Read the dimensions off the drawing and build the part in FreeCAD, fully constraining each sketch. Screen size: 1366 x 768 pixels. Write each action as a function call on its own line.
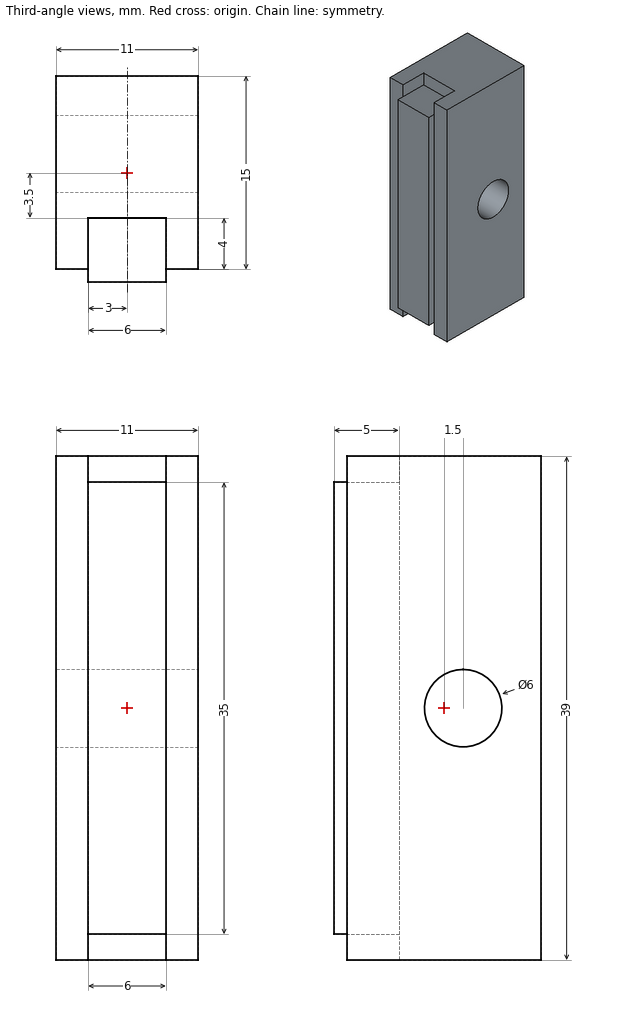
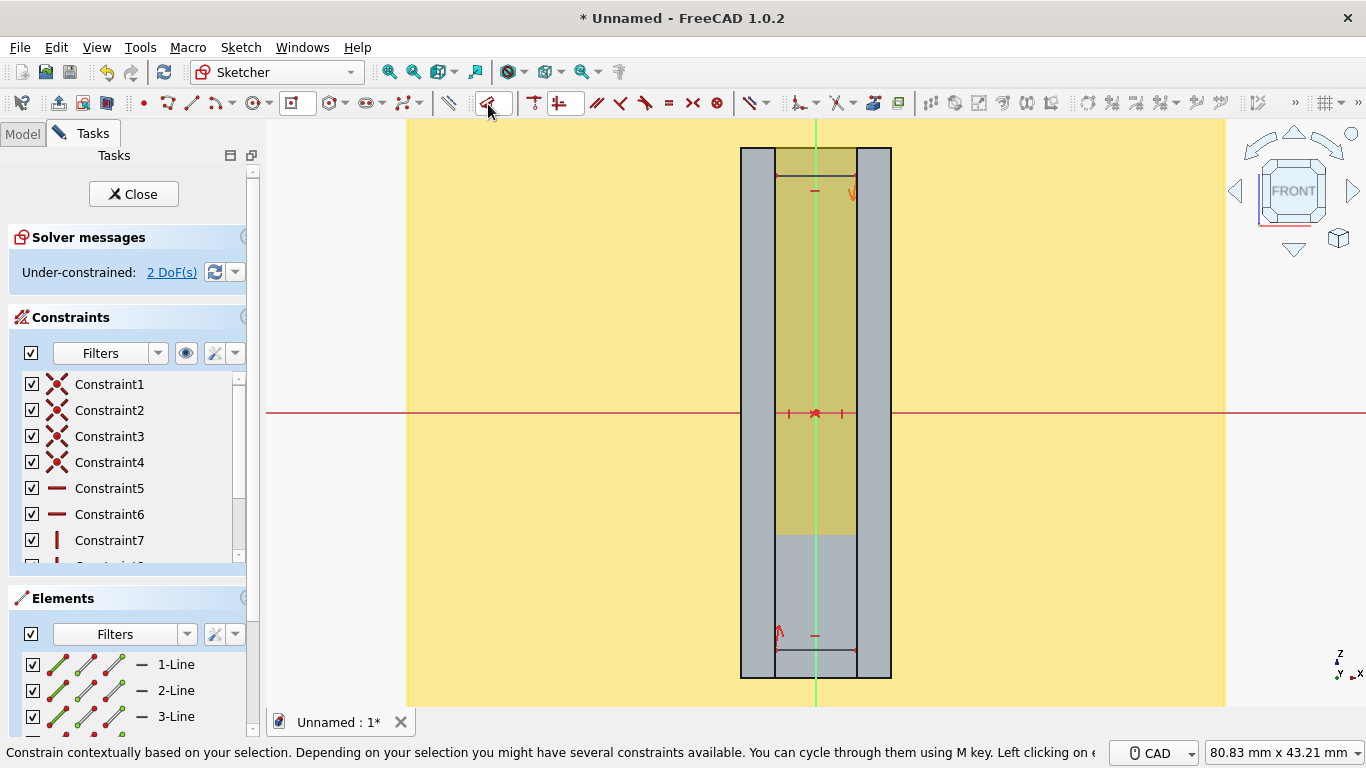
click(800, 650)
click(797, 616)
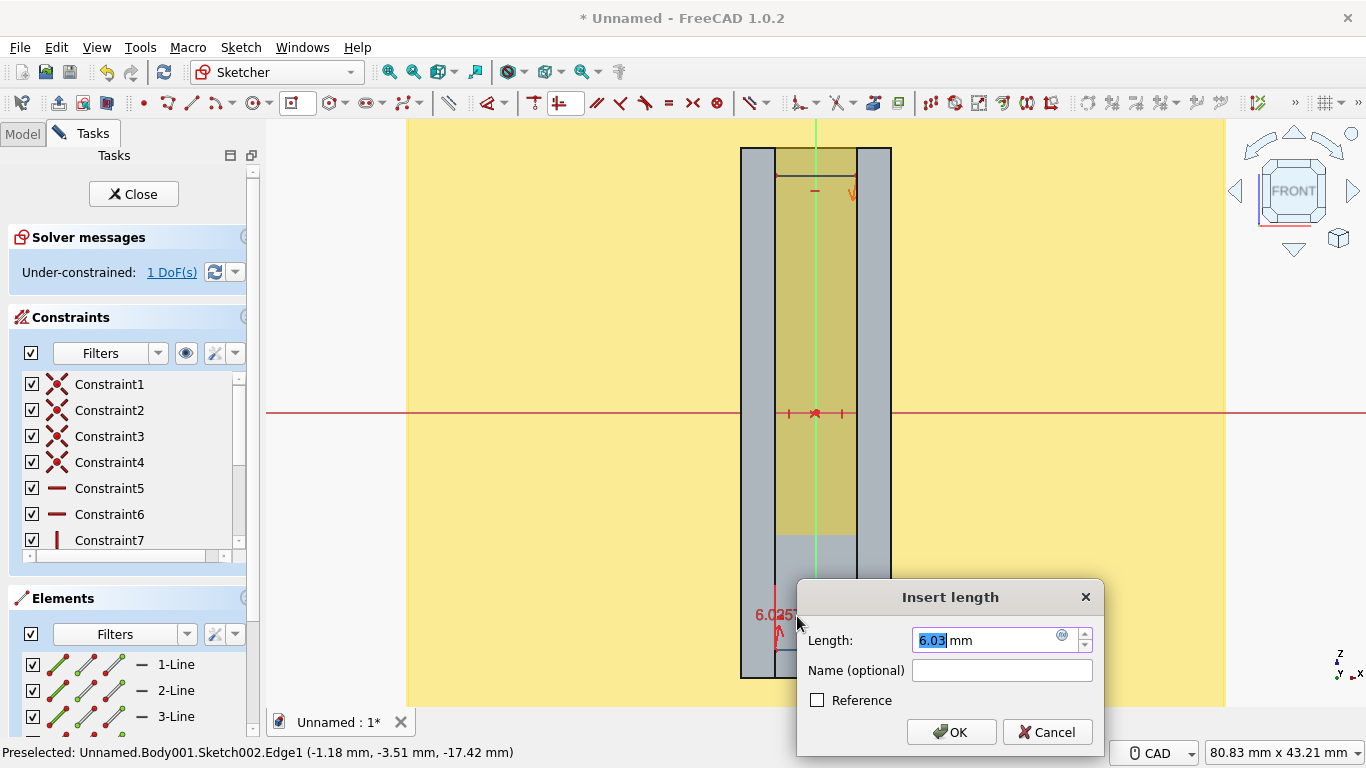
text(6)
key(Return)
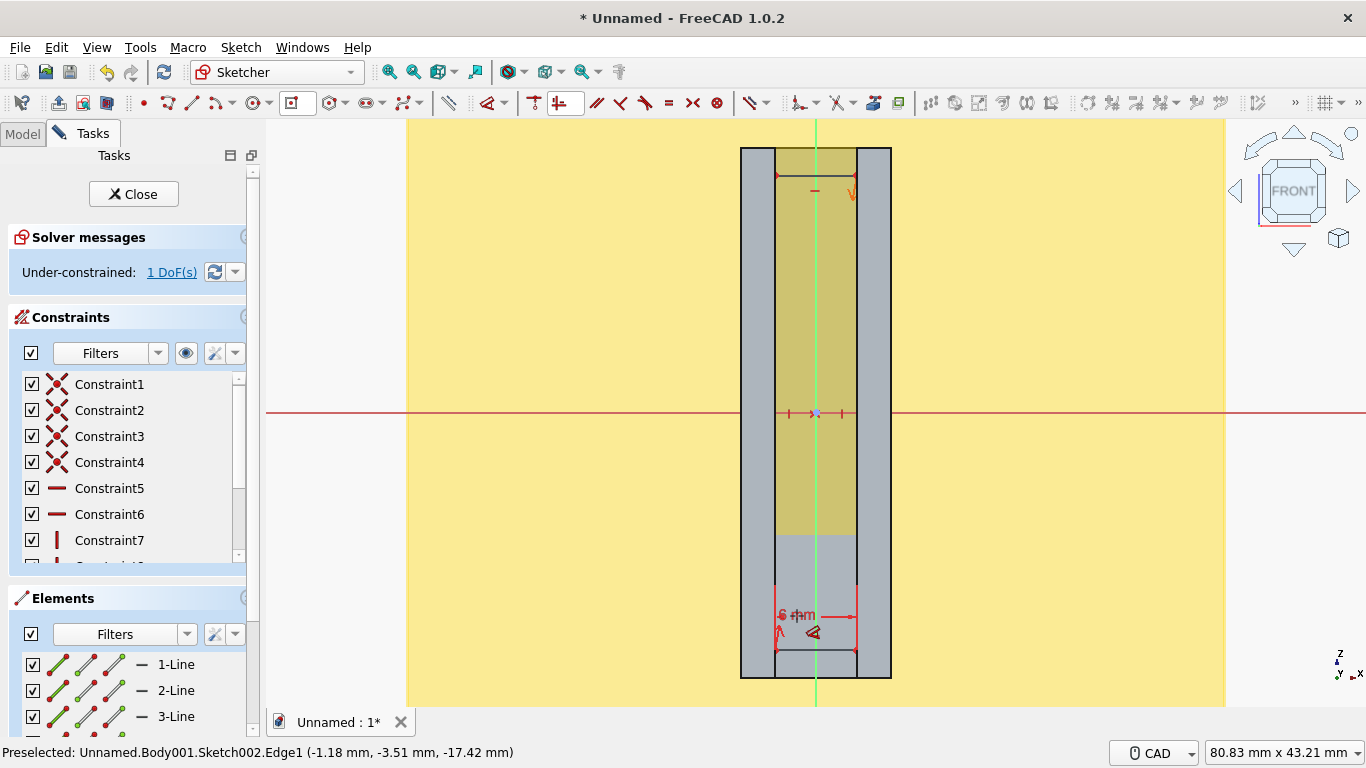
click(857, 508)
click(891, 304)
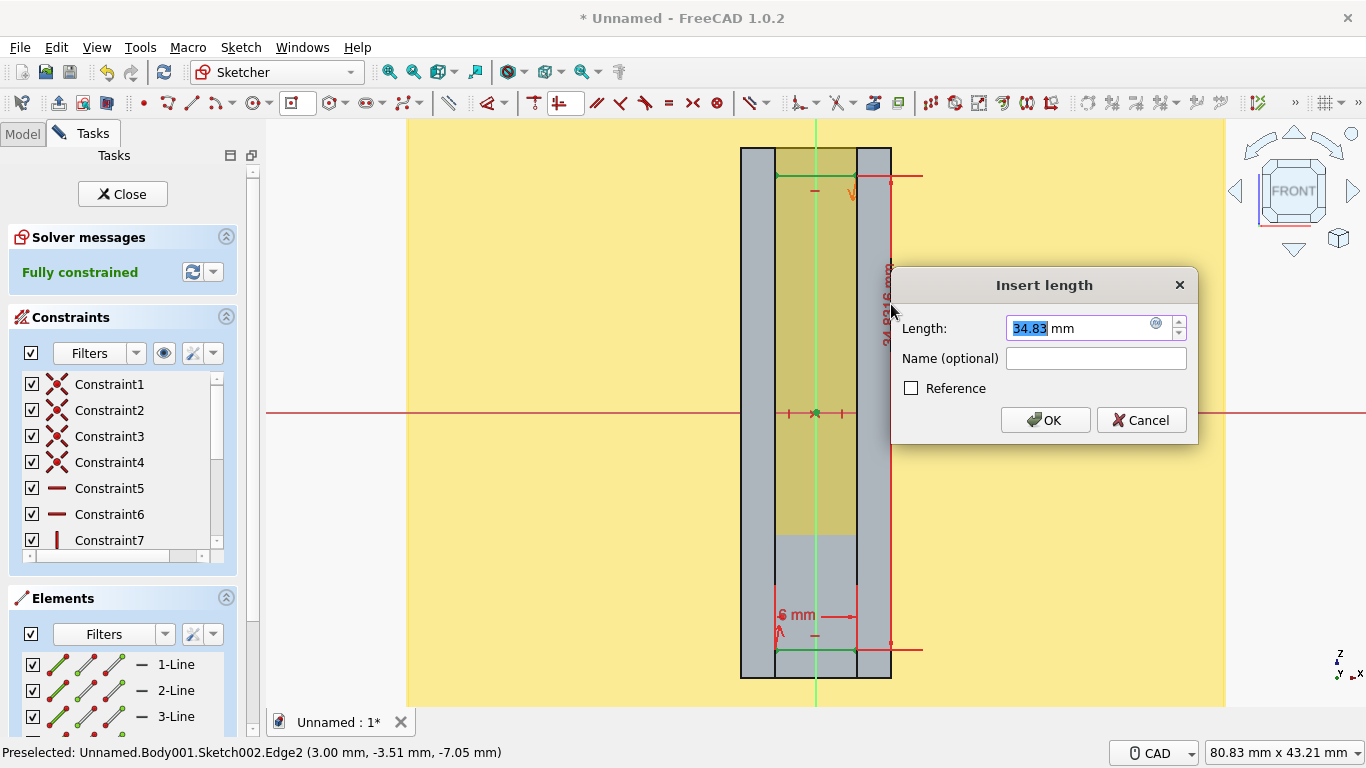
text(35)
key(Return)
key(Escape)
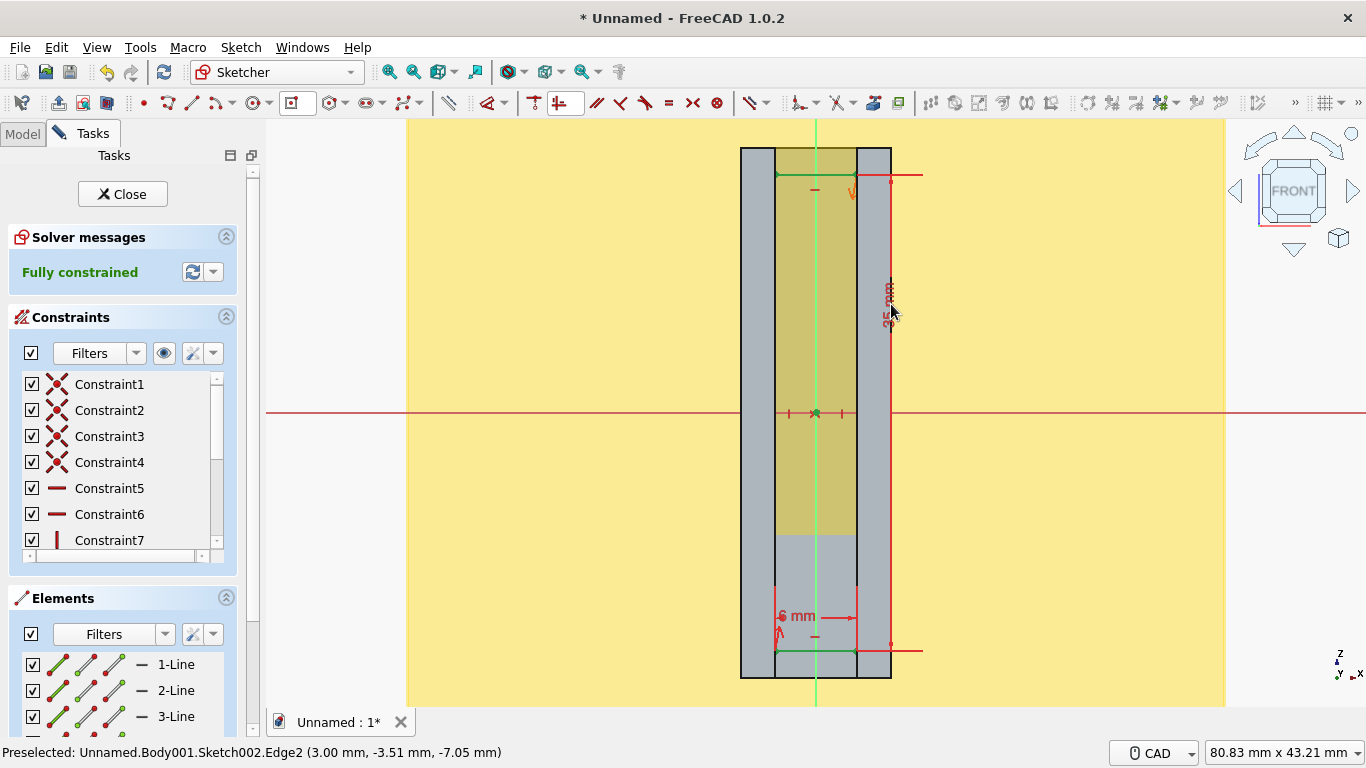
click(123, 194)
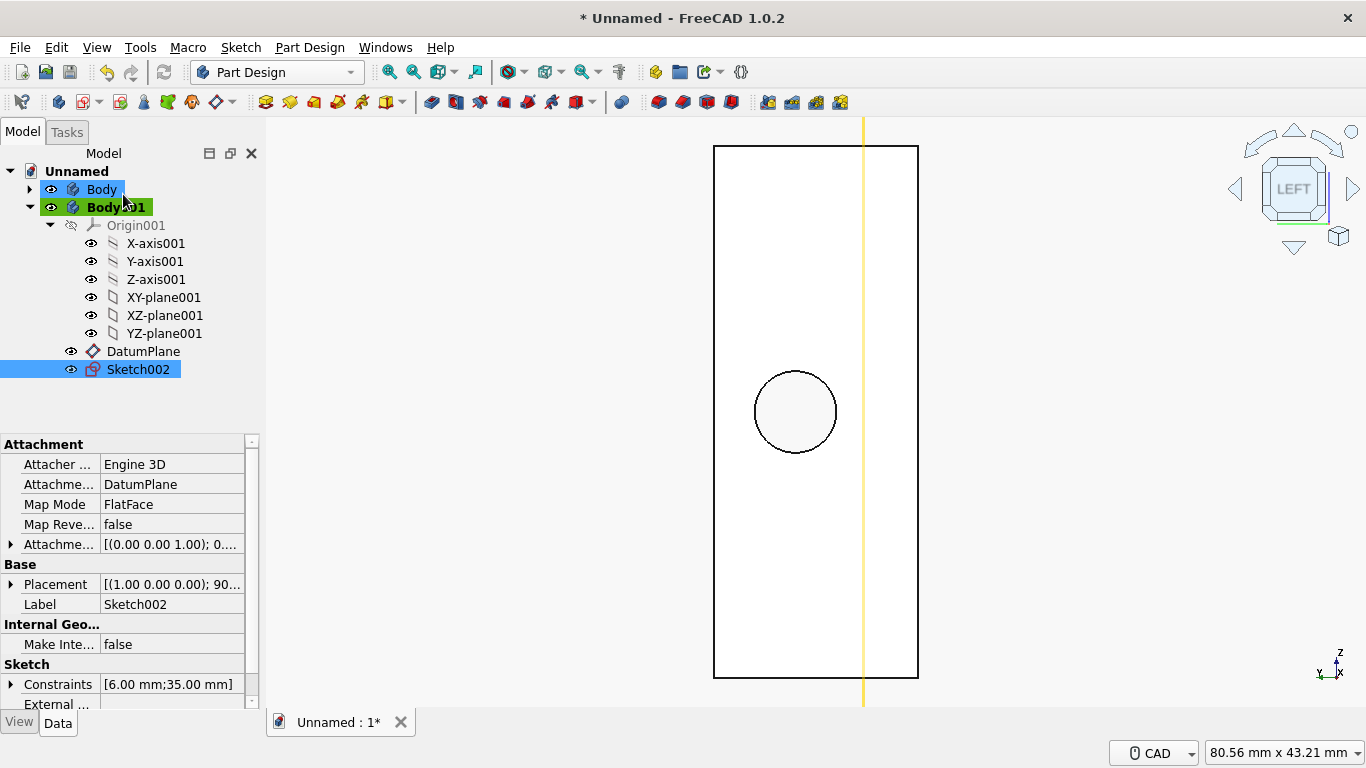
click(266, 102)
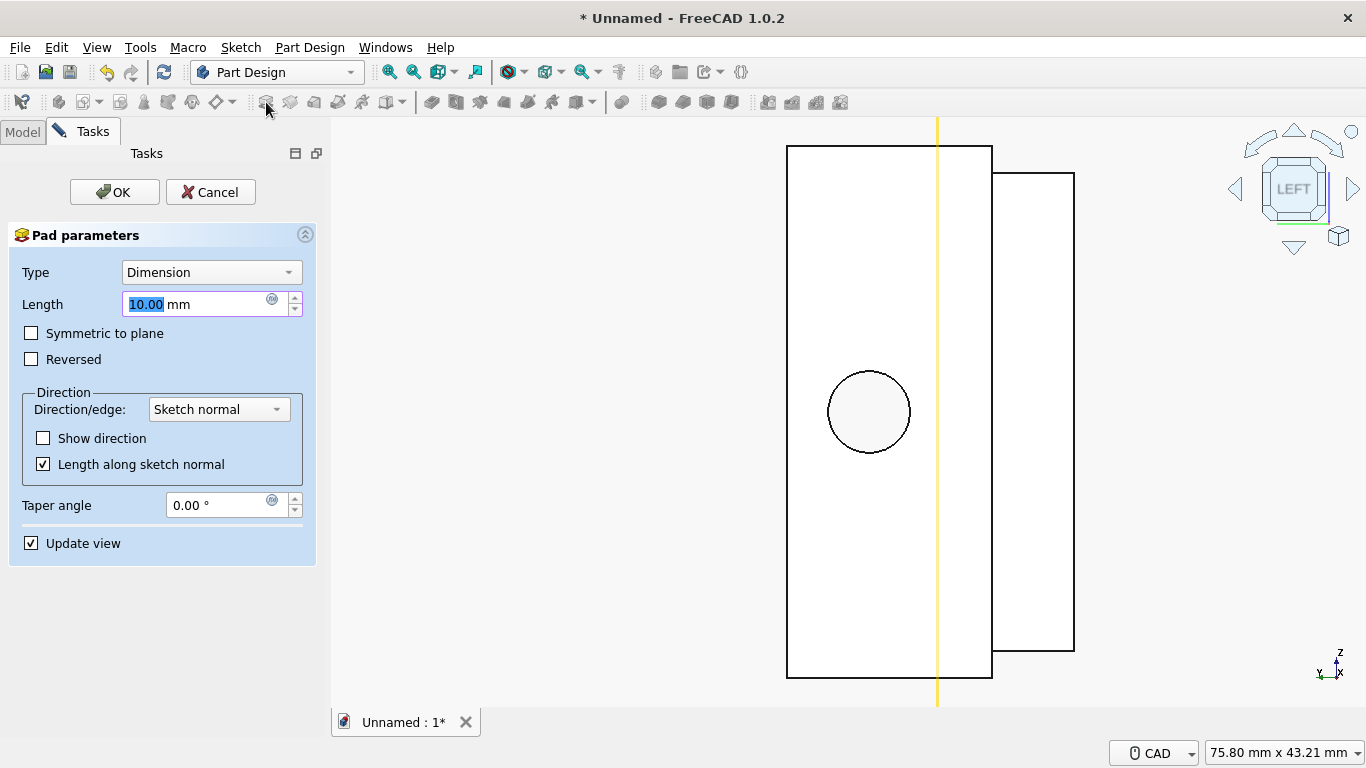
text(5)
key(Tab)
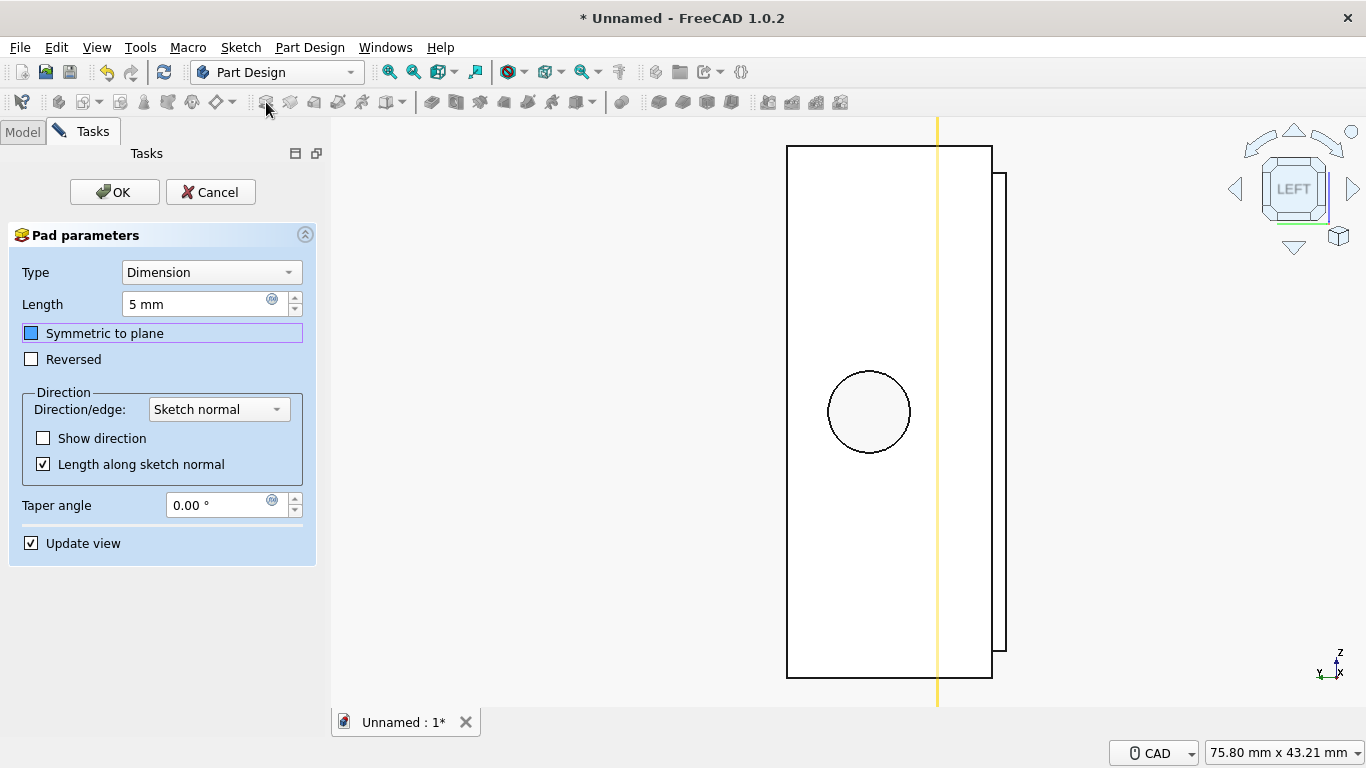
click(115, 192)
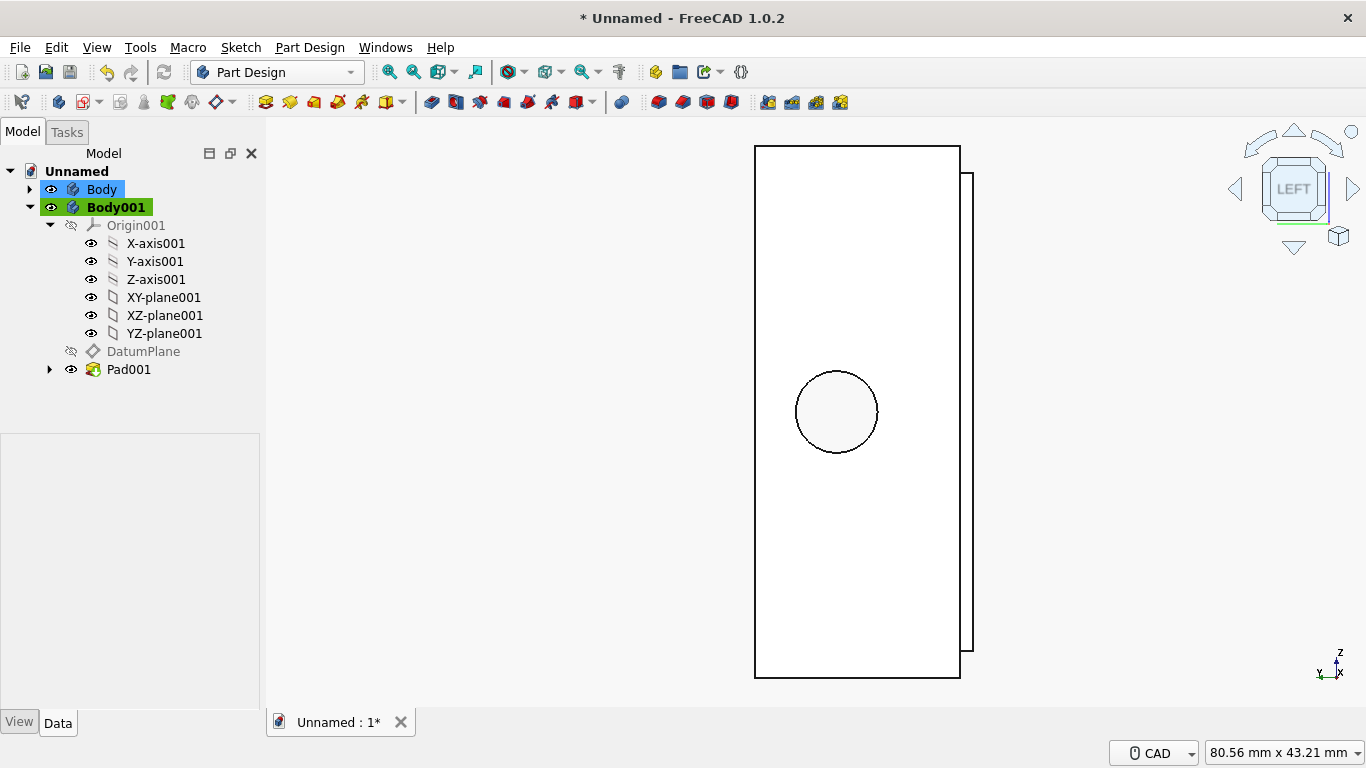
key(0)